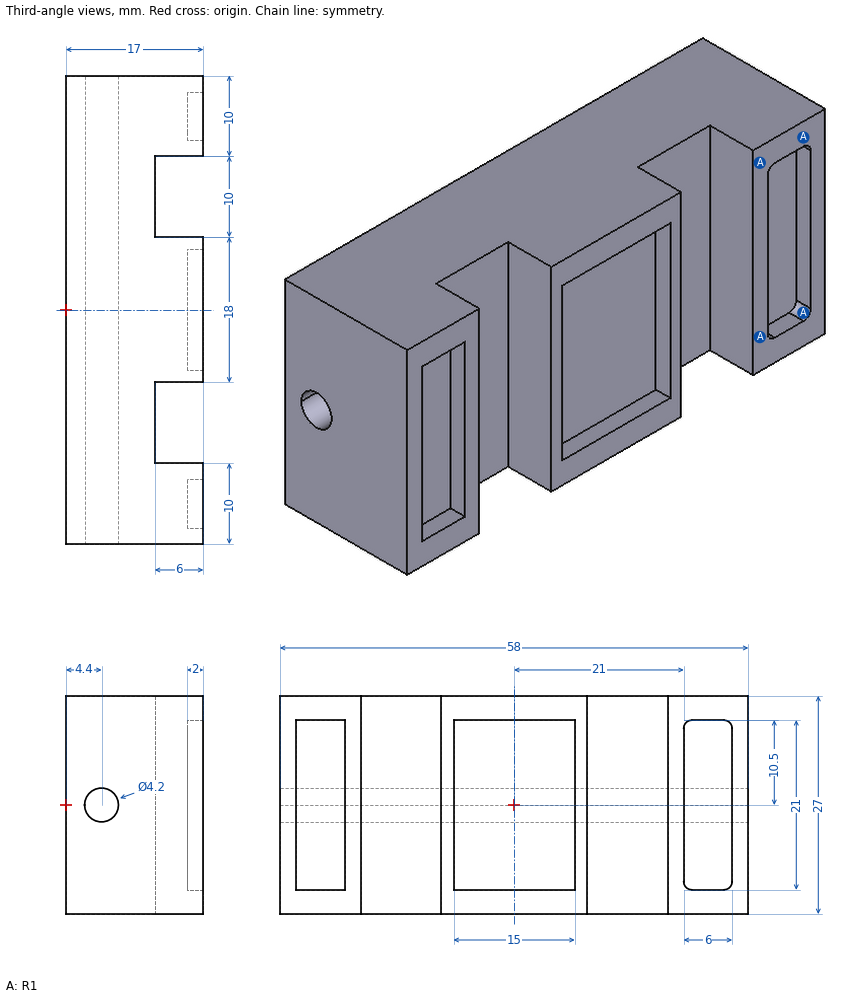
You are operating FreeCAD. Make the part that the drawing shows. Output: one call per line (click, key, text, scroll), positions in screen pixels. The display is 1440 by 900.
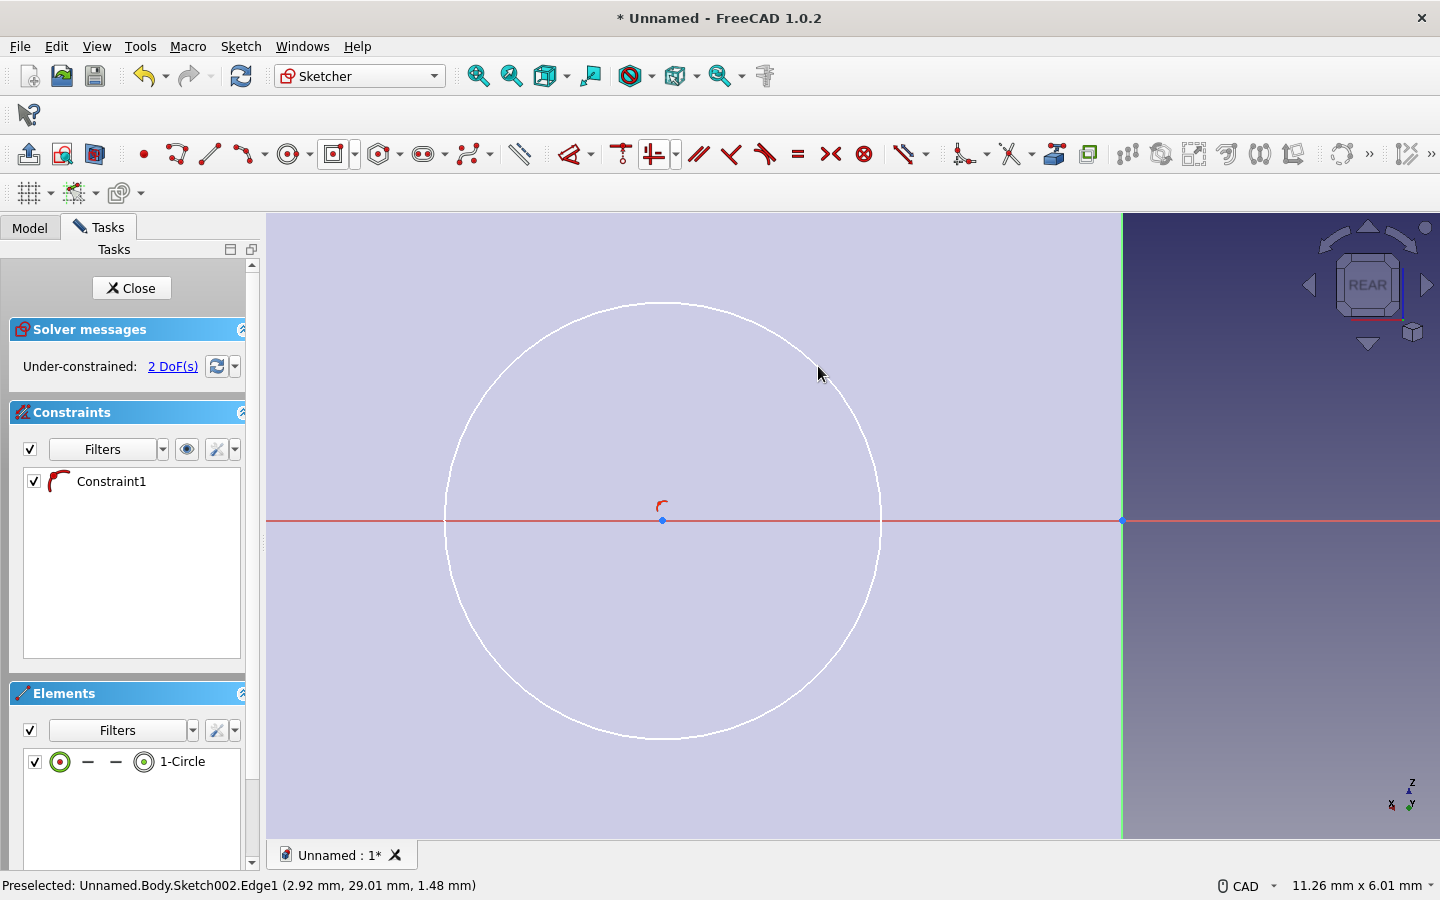
key(d)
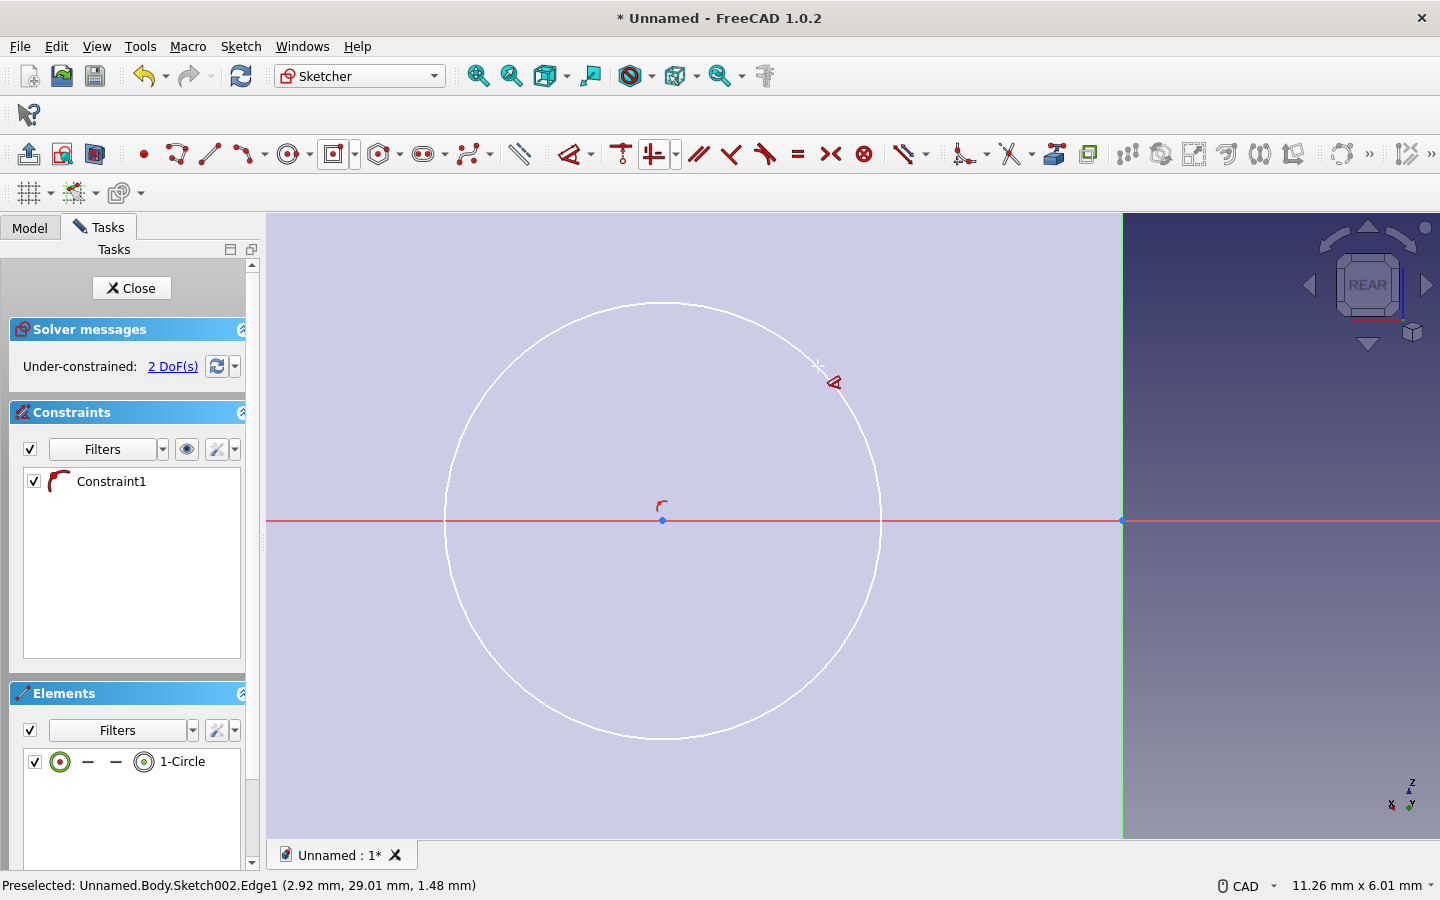
click(817, 366)
click(840, 343)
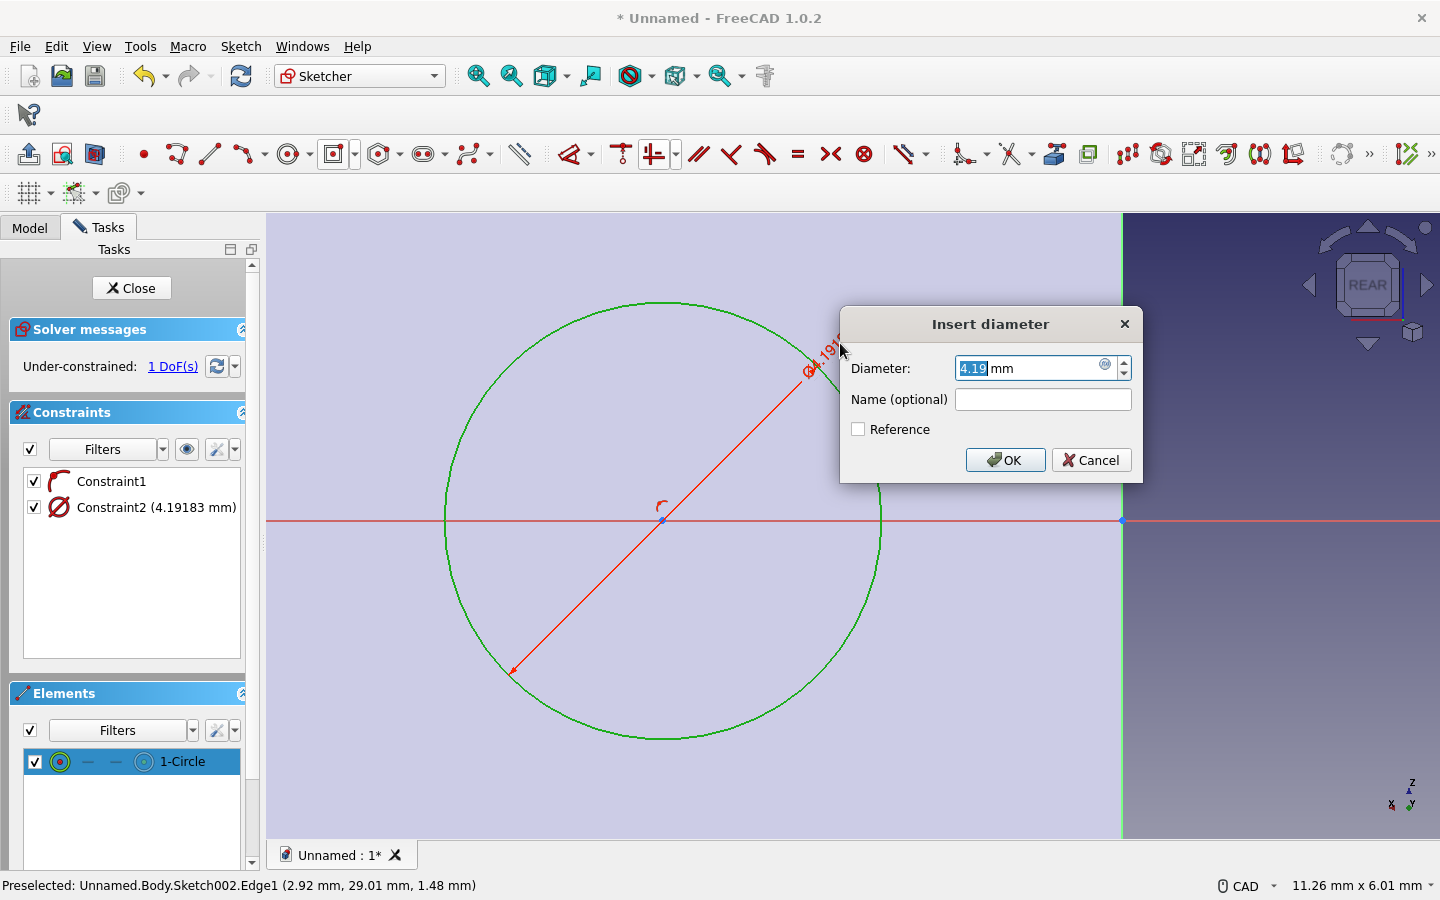
text(4.2)
key(Return)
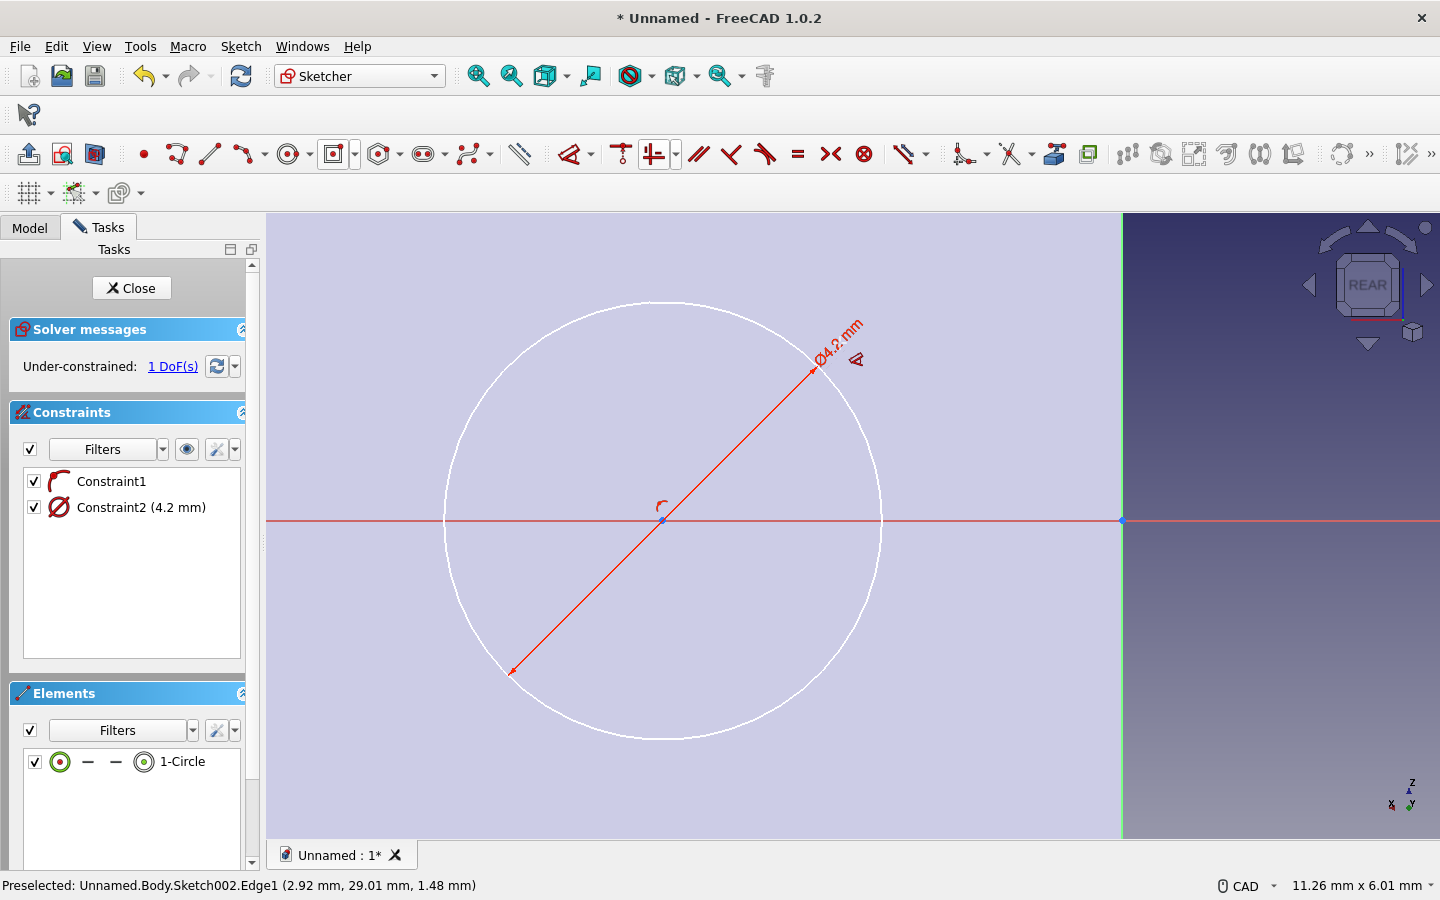
click(663, 521)
click(893, 555)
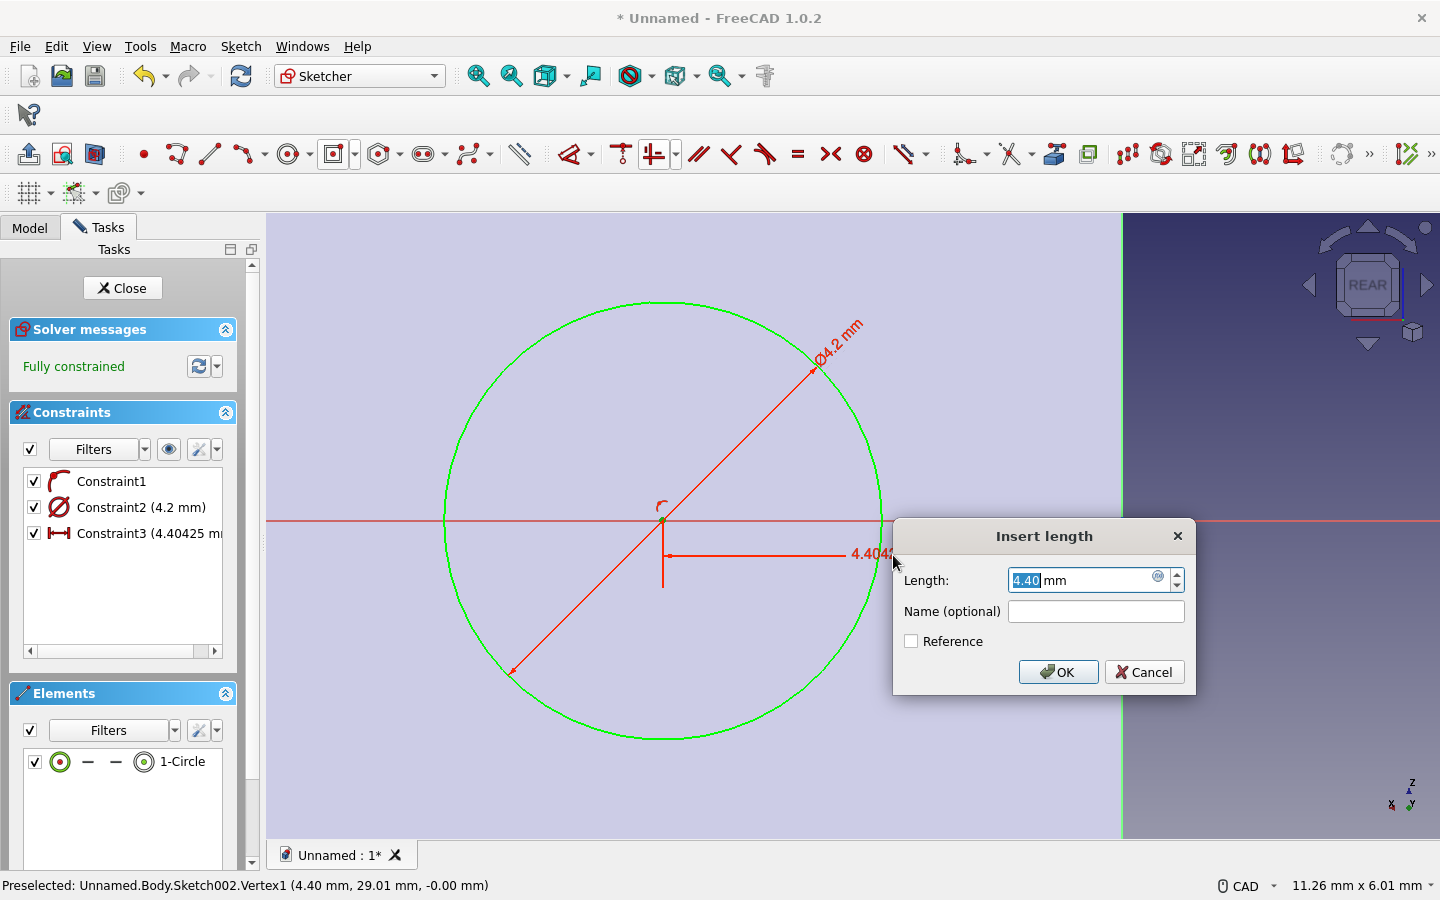
text(4.4)
key(Return)
key(Escape)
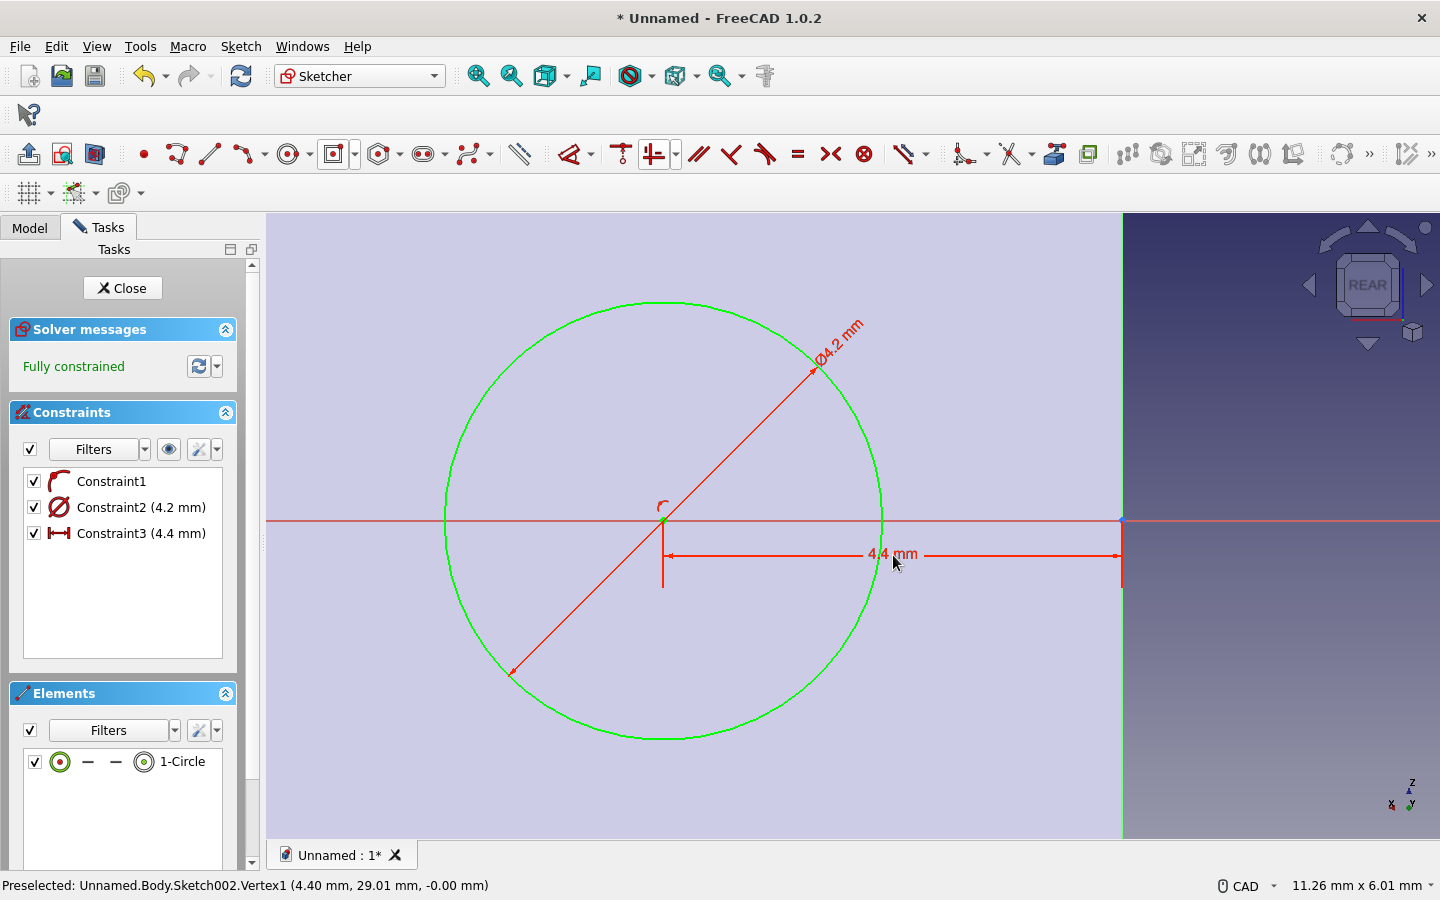
click(123, 288)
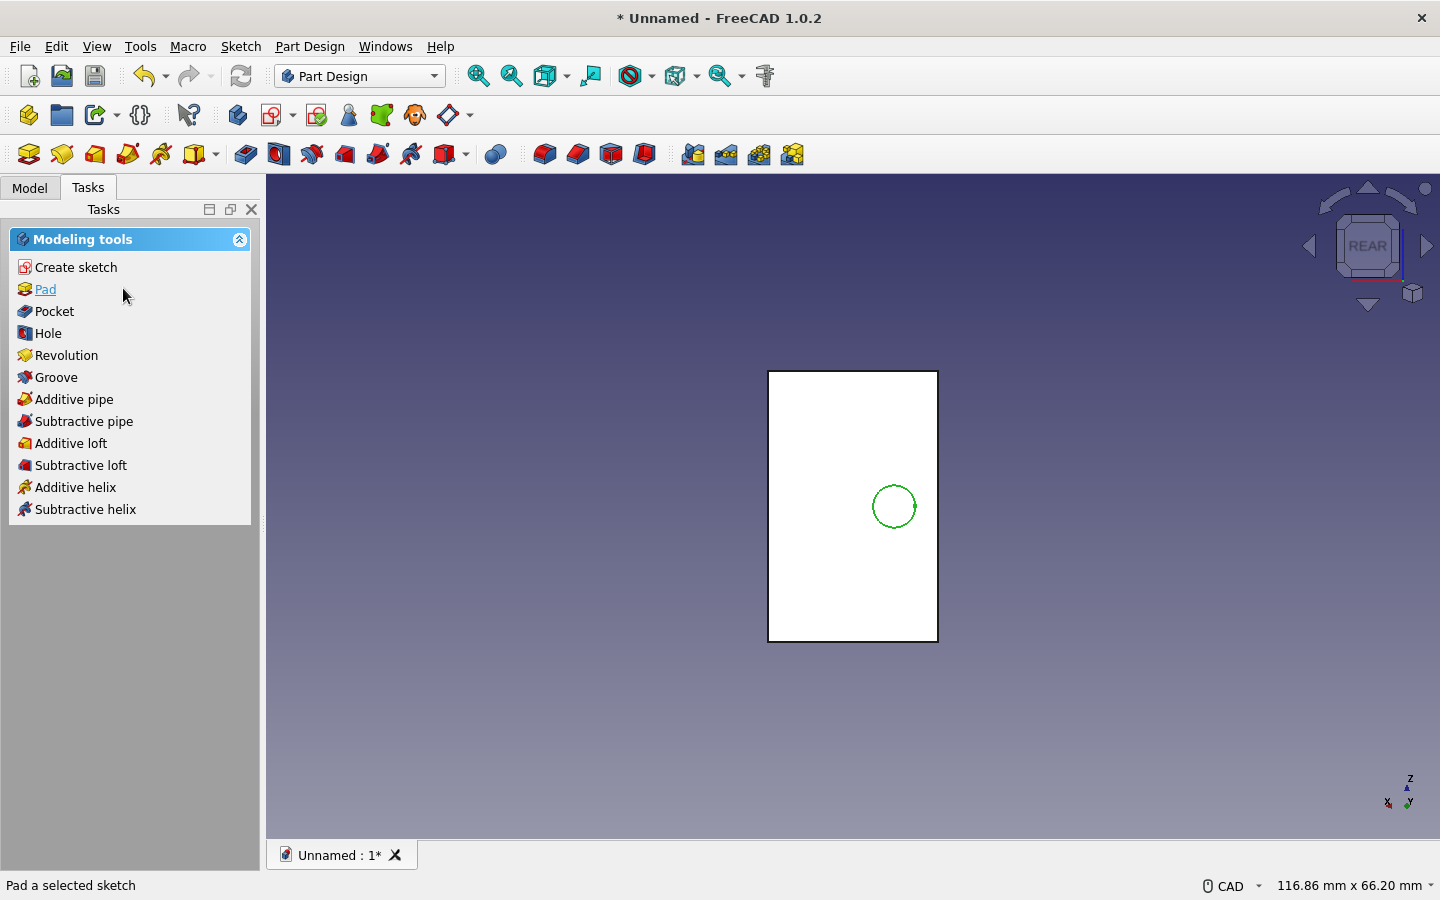
click(246, 154)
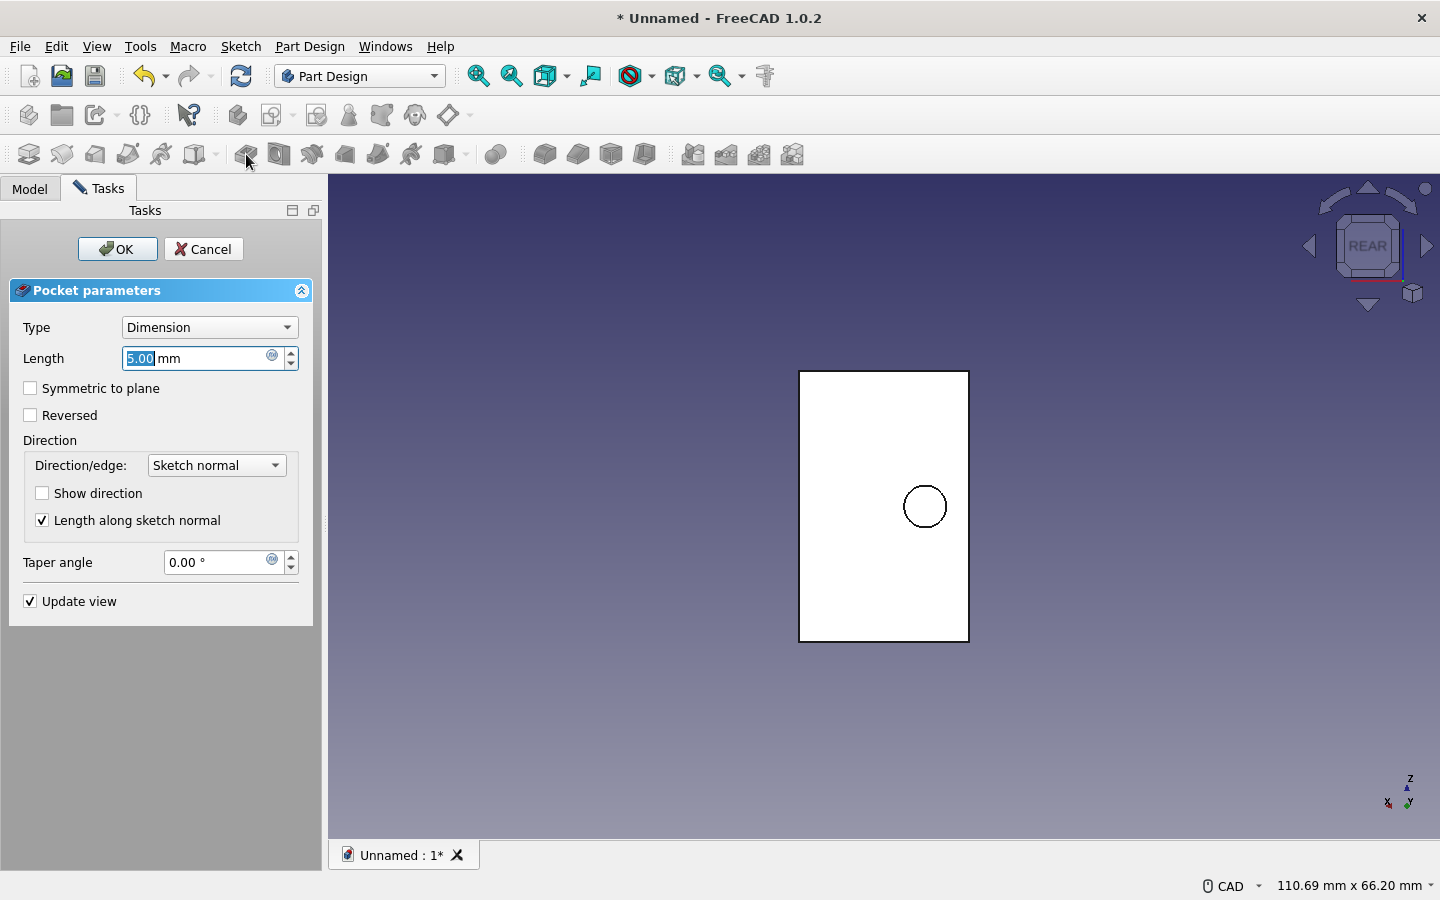
text(58)
key(Tab)